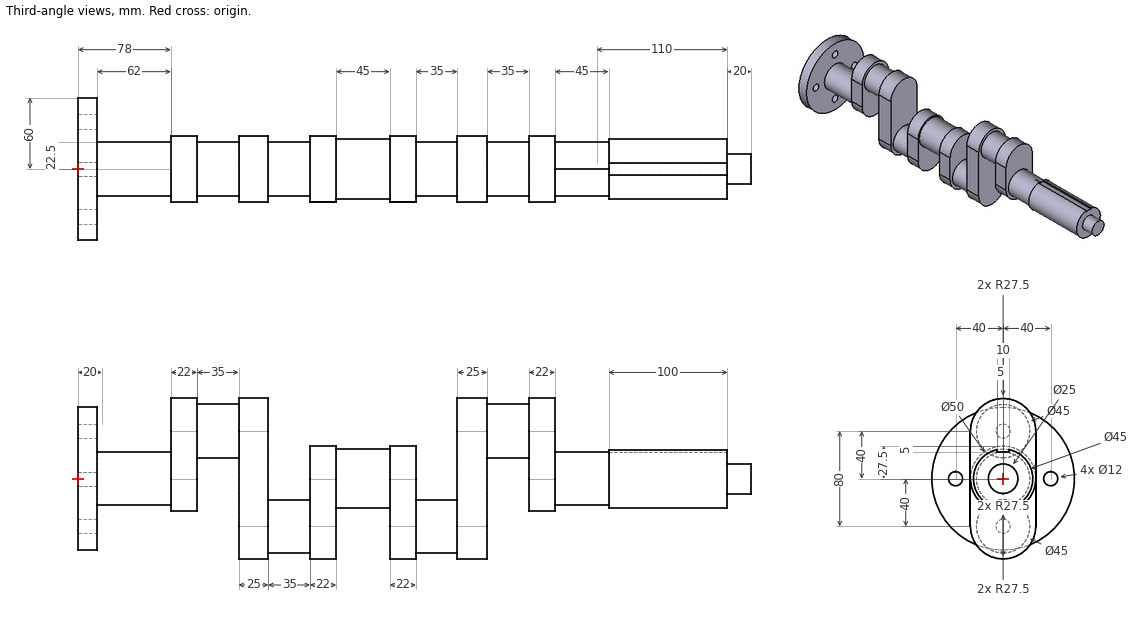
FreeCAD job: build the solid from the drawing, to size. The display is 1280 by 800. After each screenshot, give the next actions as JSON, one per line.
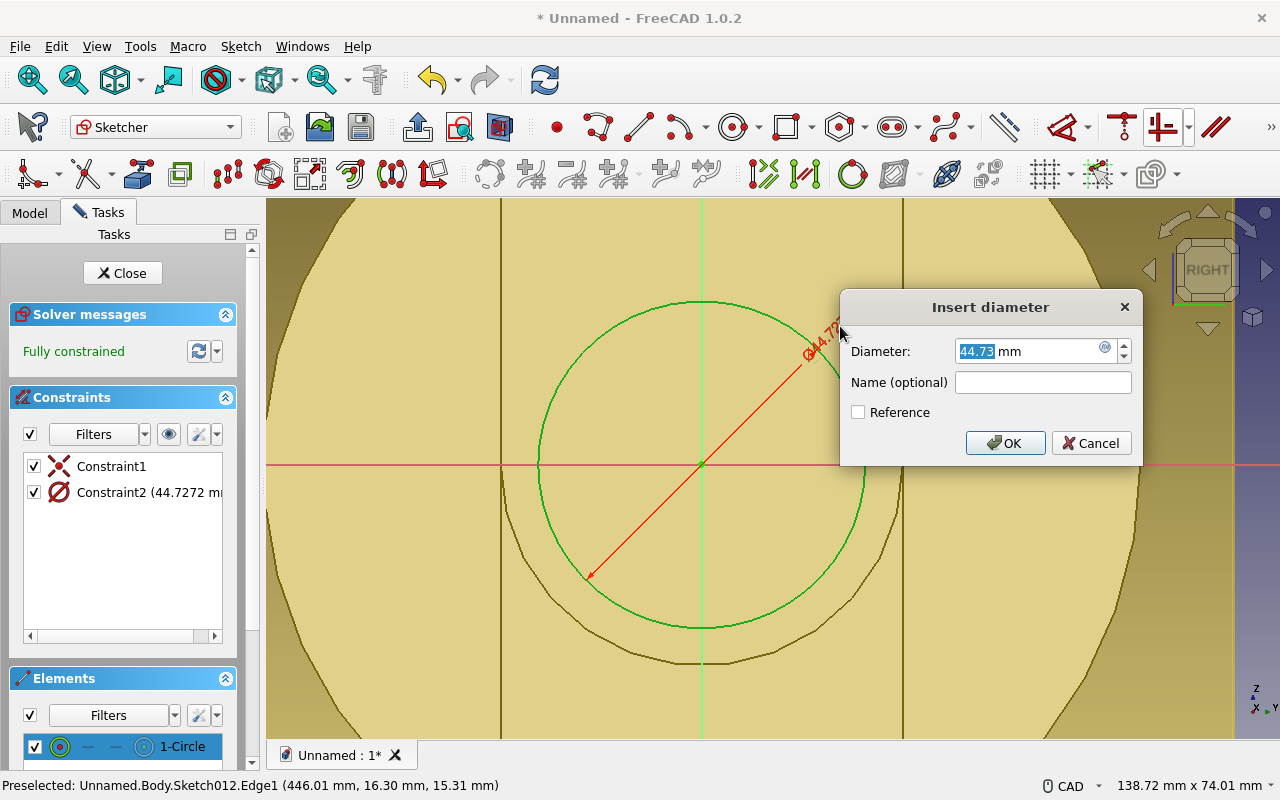
{"action": "type", "text": "45"}
{"action": "key", "text": "Return"}
{"action": "key", "text": "Escape"}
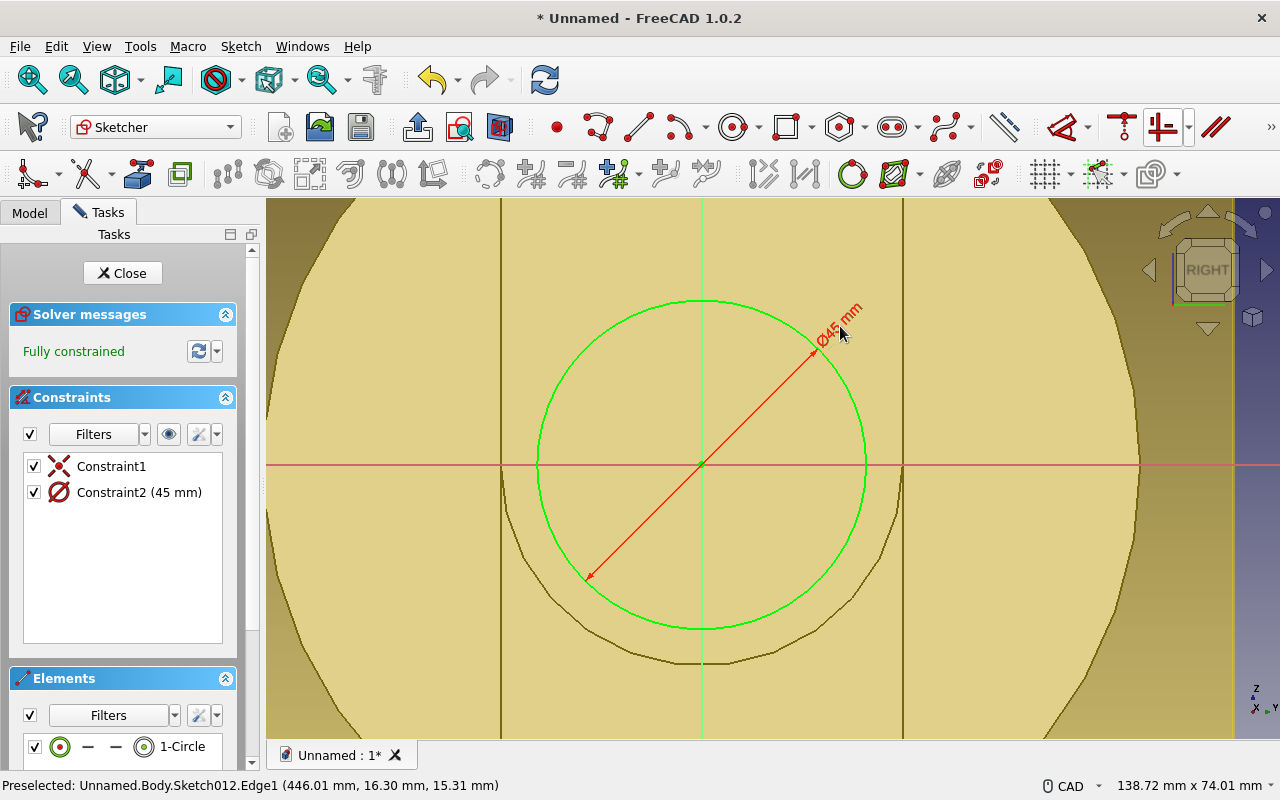
{"action": "left_click", "coordinate": [123, 273]}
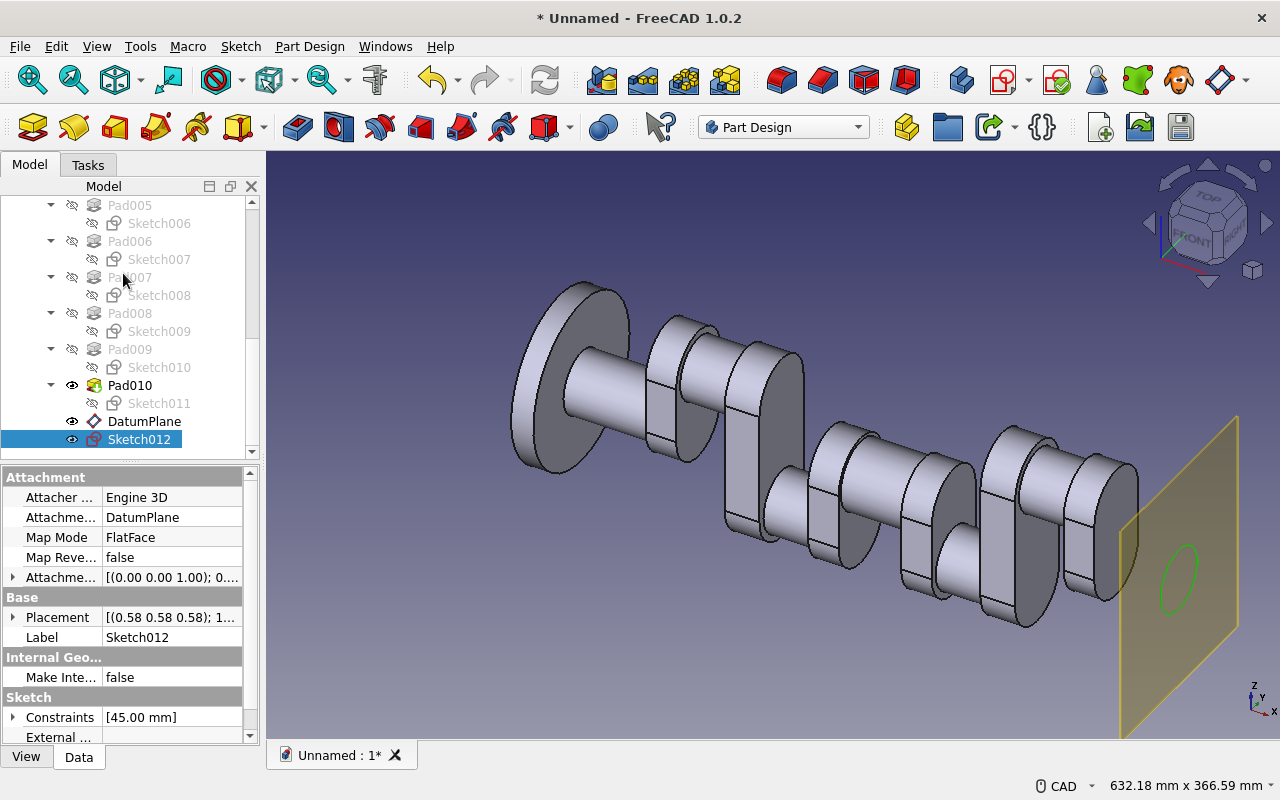
{"action": "left_click", "coordinate": [33, 128]}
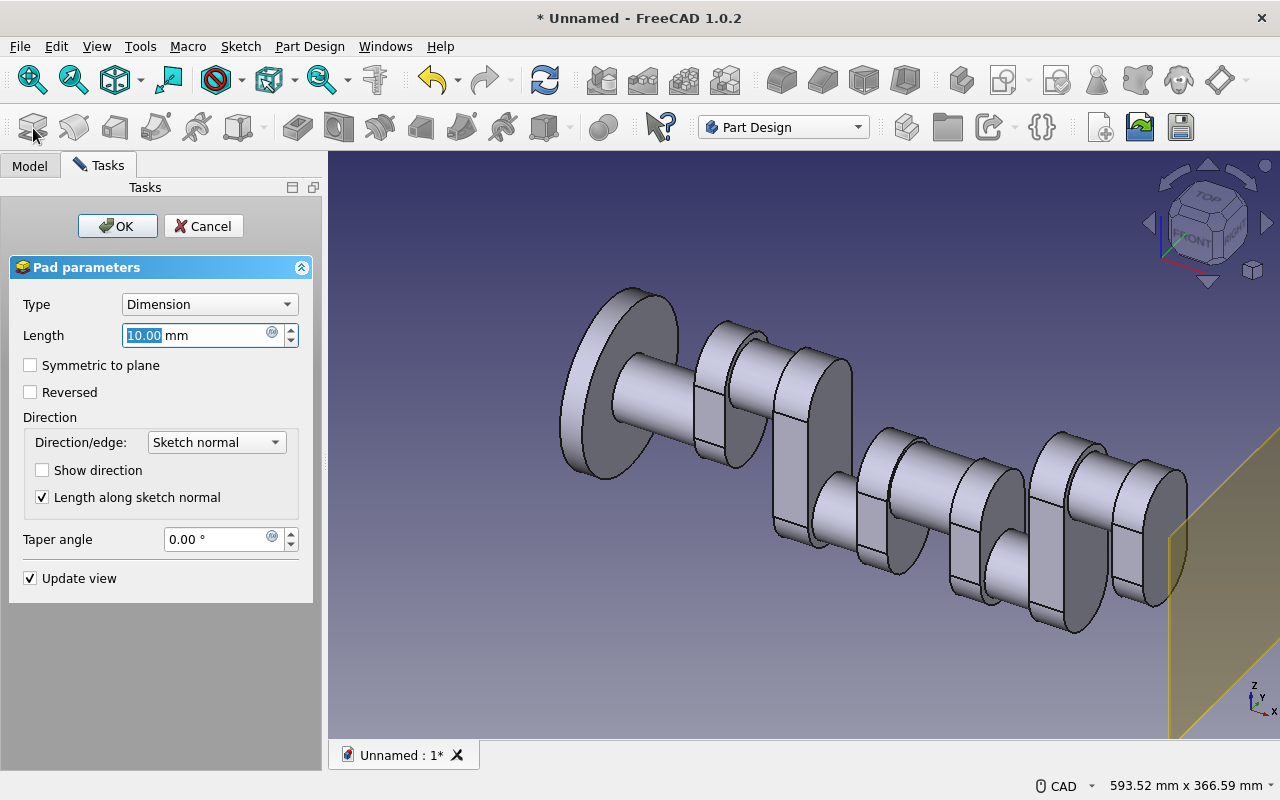
{"action": "type", "text": "45"}
{"action": "key", "text": "Tab"}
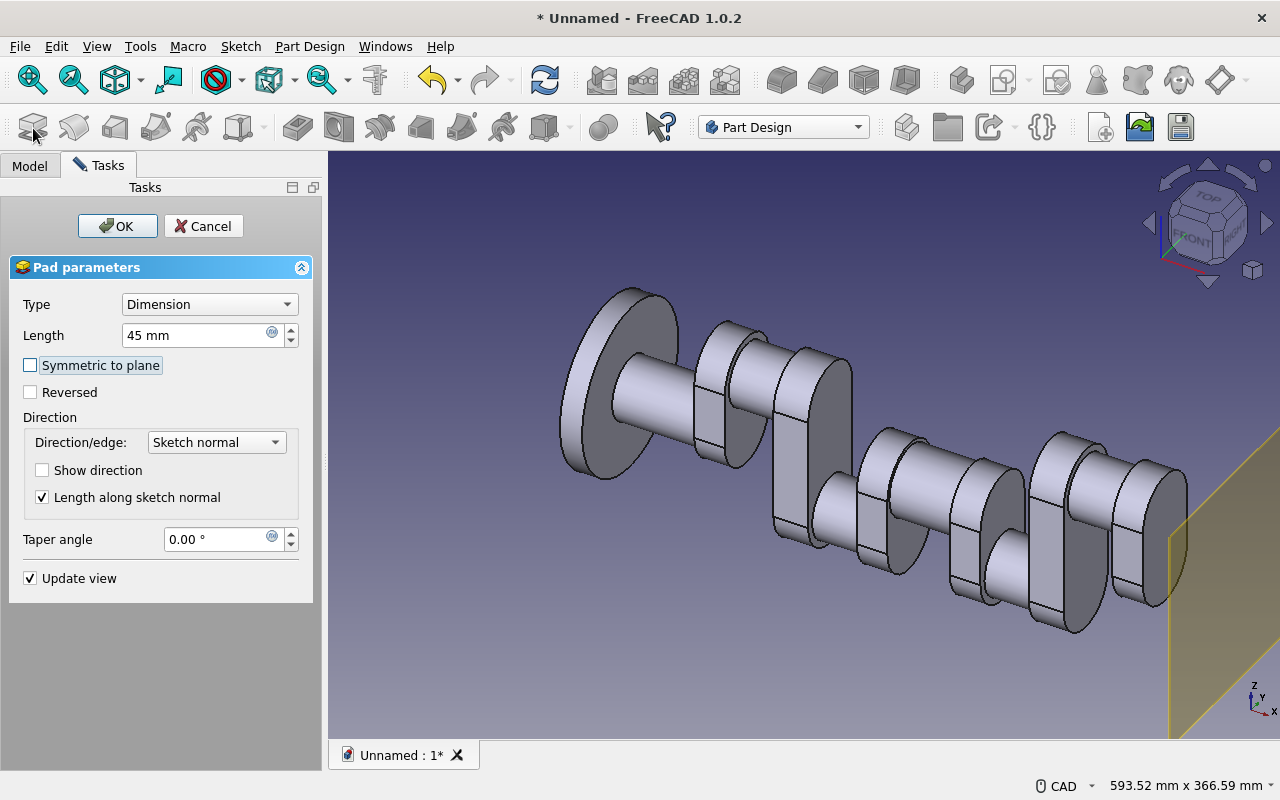
{"action": "left_click", "coordinate": [31, 392]}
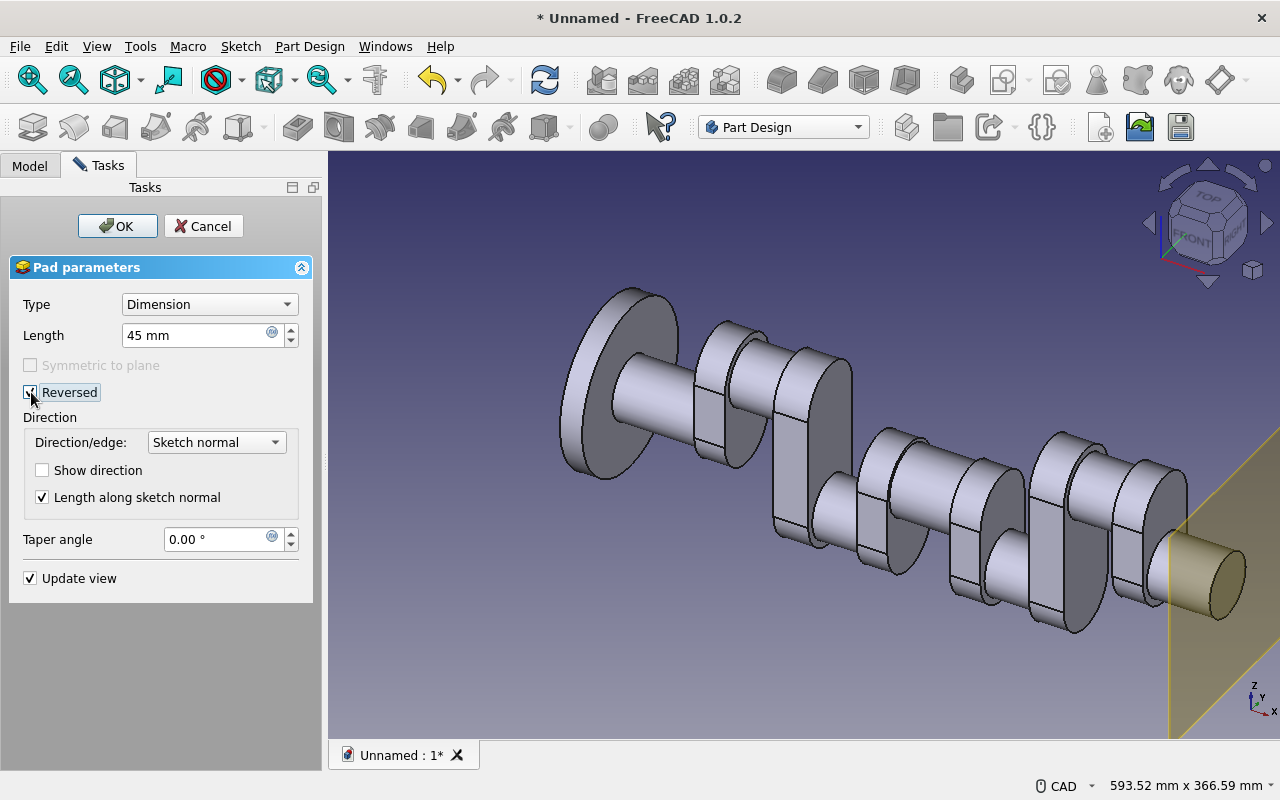
{"action": "left_click", "coordinate": [118, 226]}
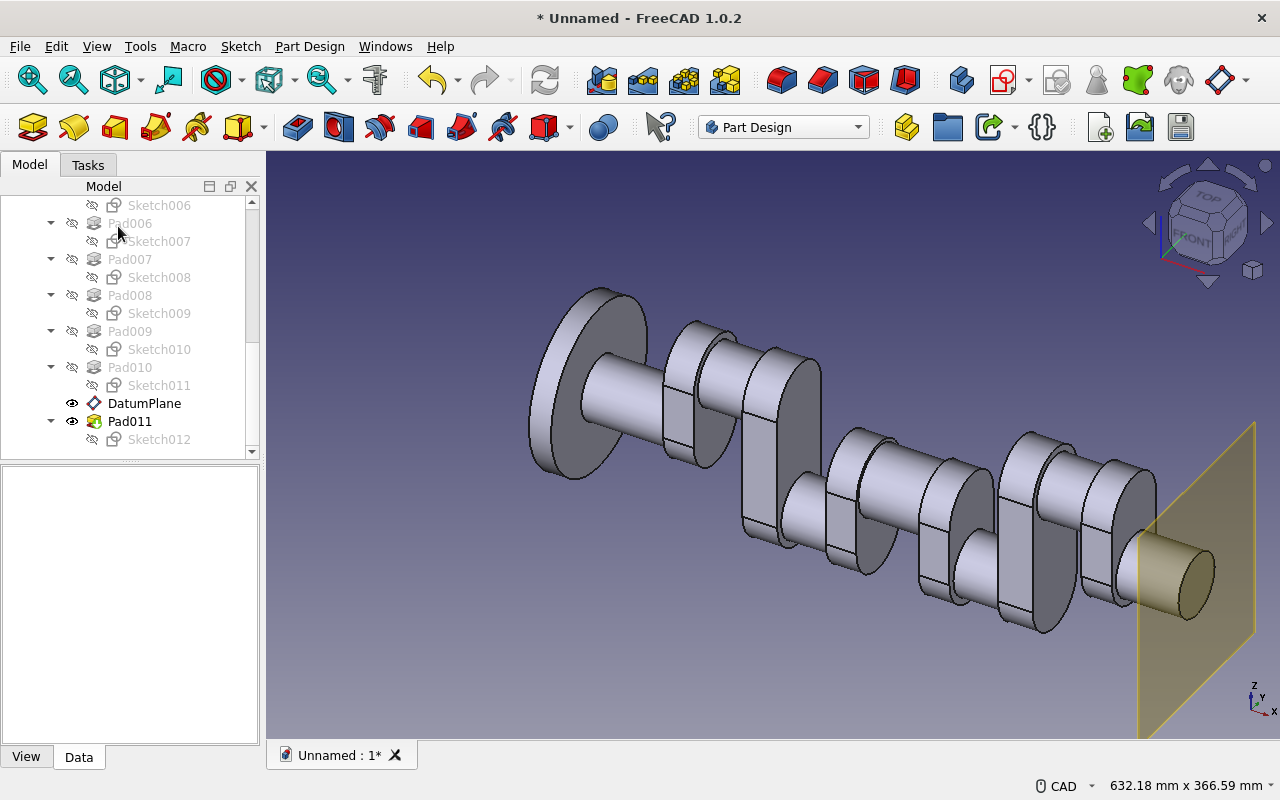
{"action": "left_click", "coordinate": [117, 403]}
{"action": "key", "text": "space"}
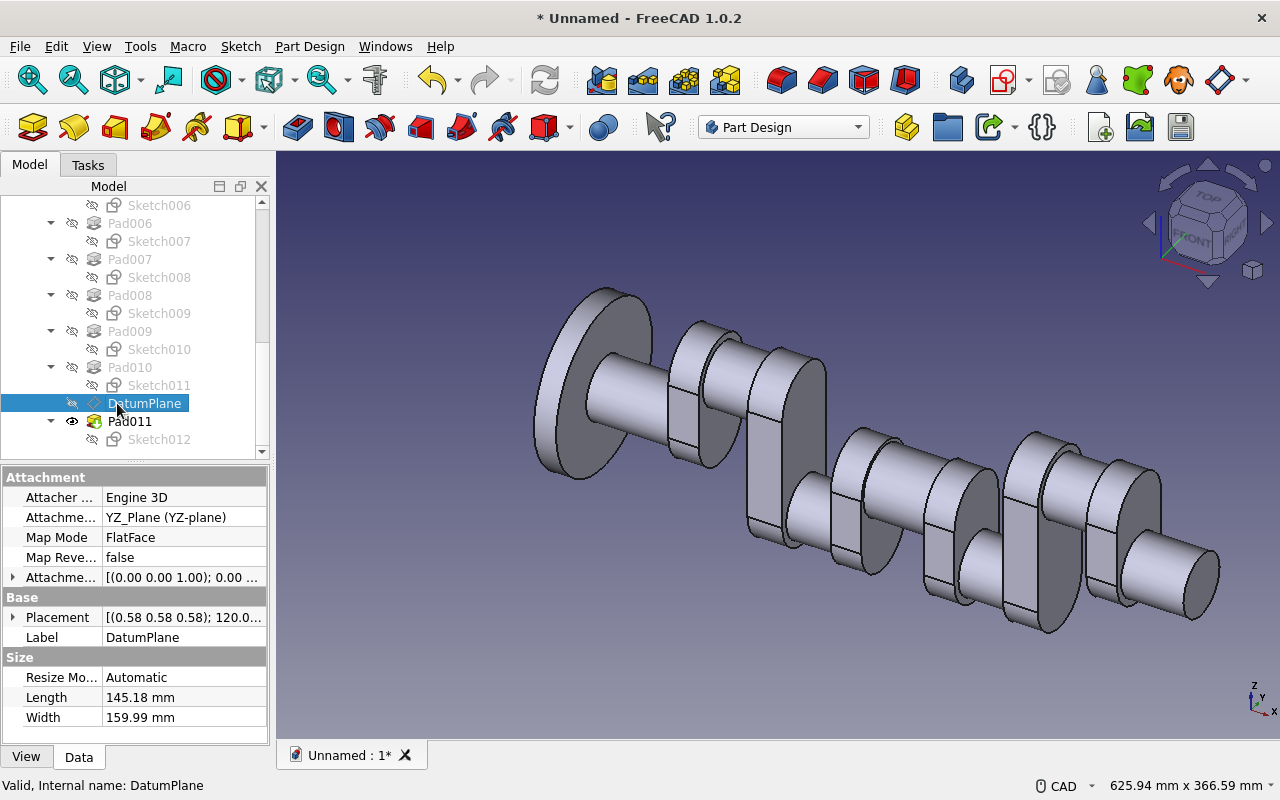
{"action": "left_click", "coordinate": [1202, 584]}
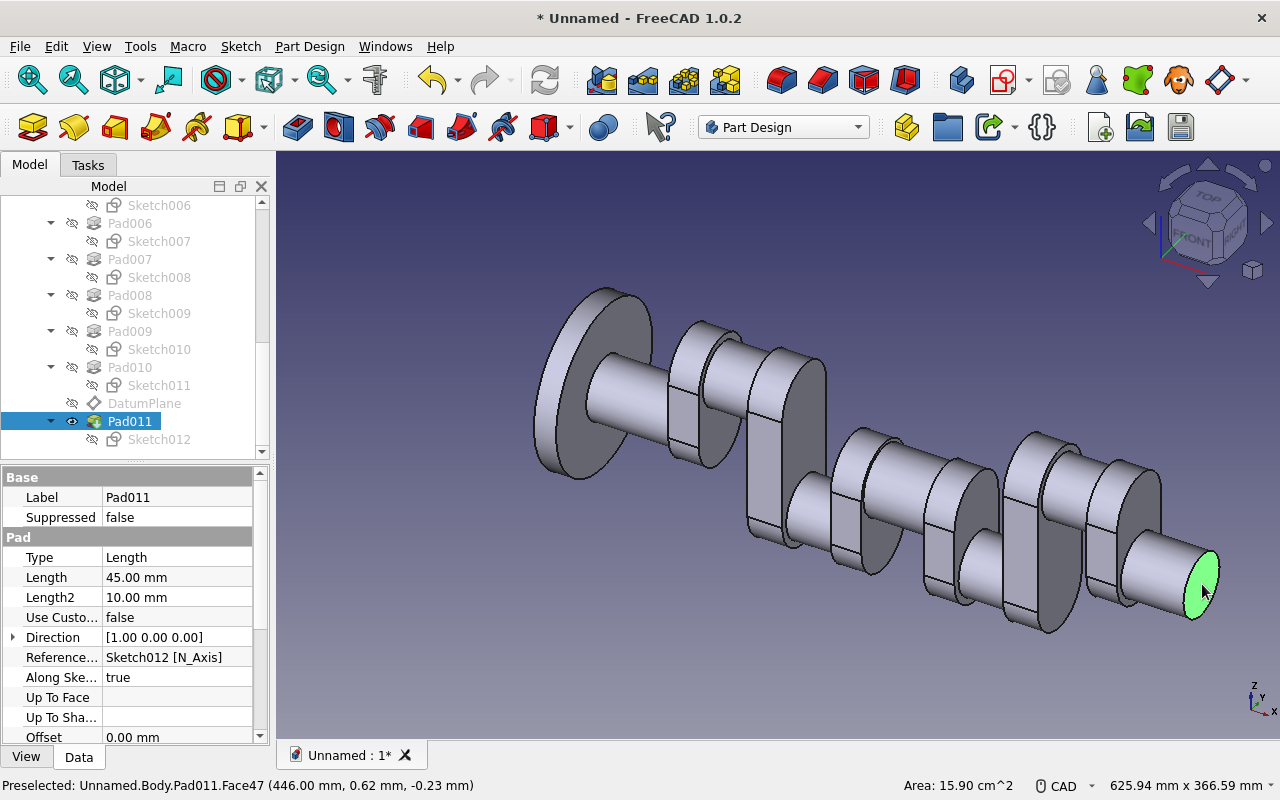
{"action": "left_click", "coordinate": [1002, 80]}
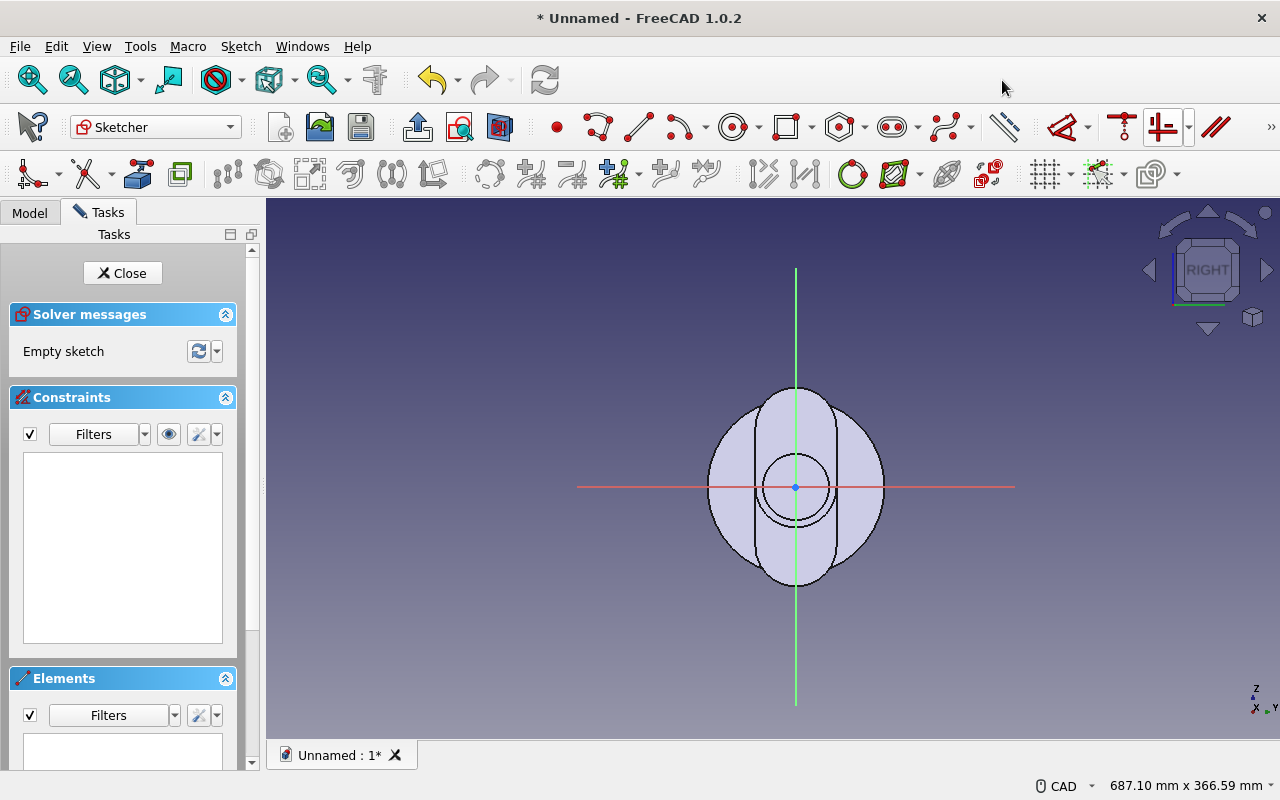
{"action": "scroll", "coordinate": [819, 492], "scroll_direction": "up", "scroll_amount": 8}